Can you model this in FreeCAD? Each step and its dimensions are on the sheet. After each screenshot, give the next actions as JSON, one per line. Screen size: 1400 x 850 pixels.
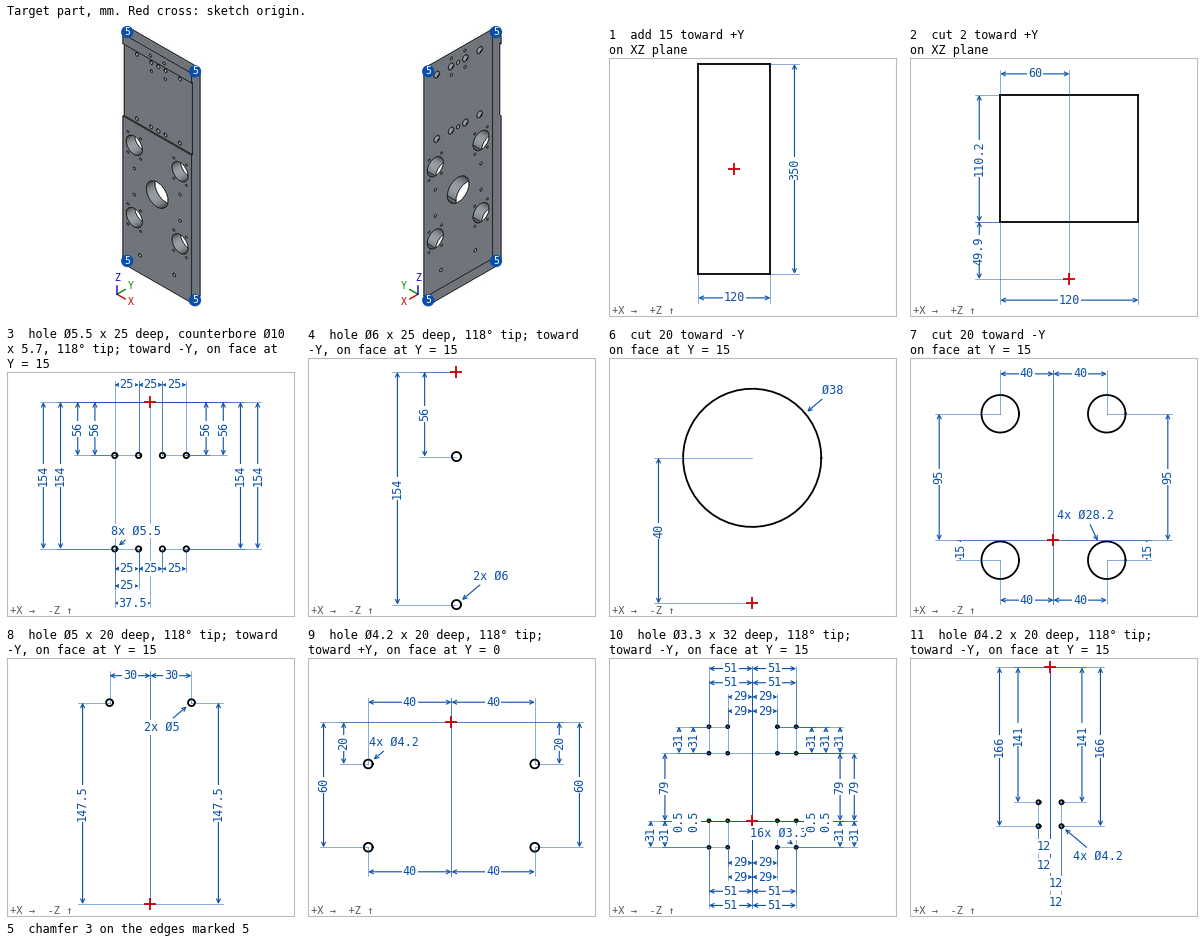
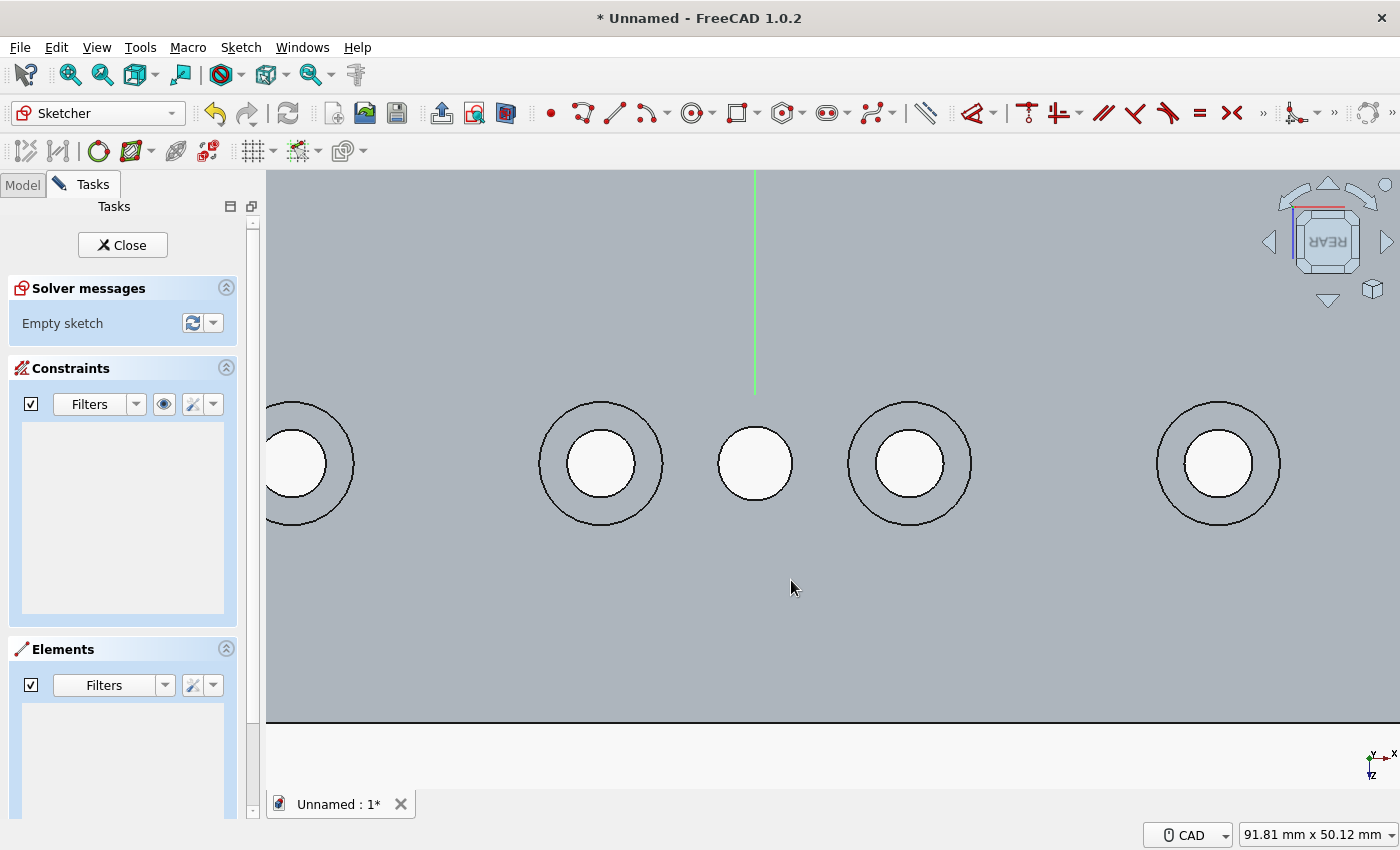
{"action": "left_click", "coordinate": [692, 114]}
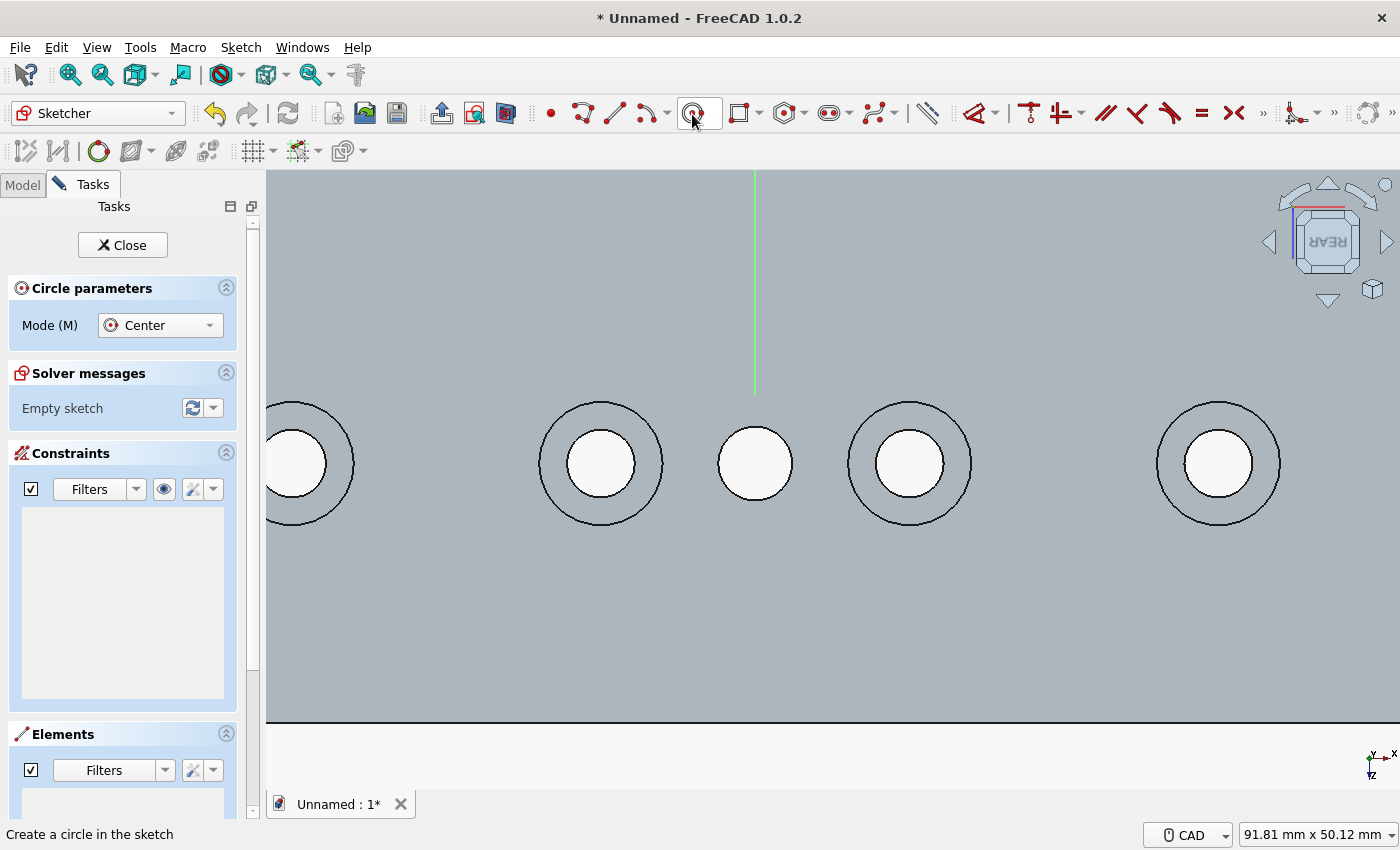
{"action": "left_click", "coordinate": [607, 303]}
{"action": "left_click", "coordinate": [625, 285]}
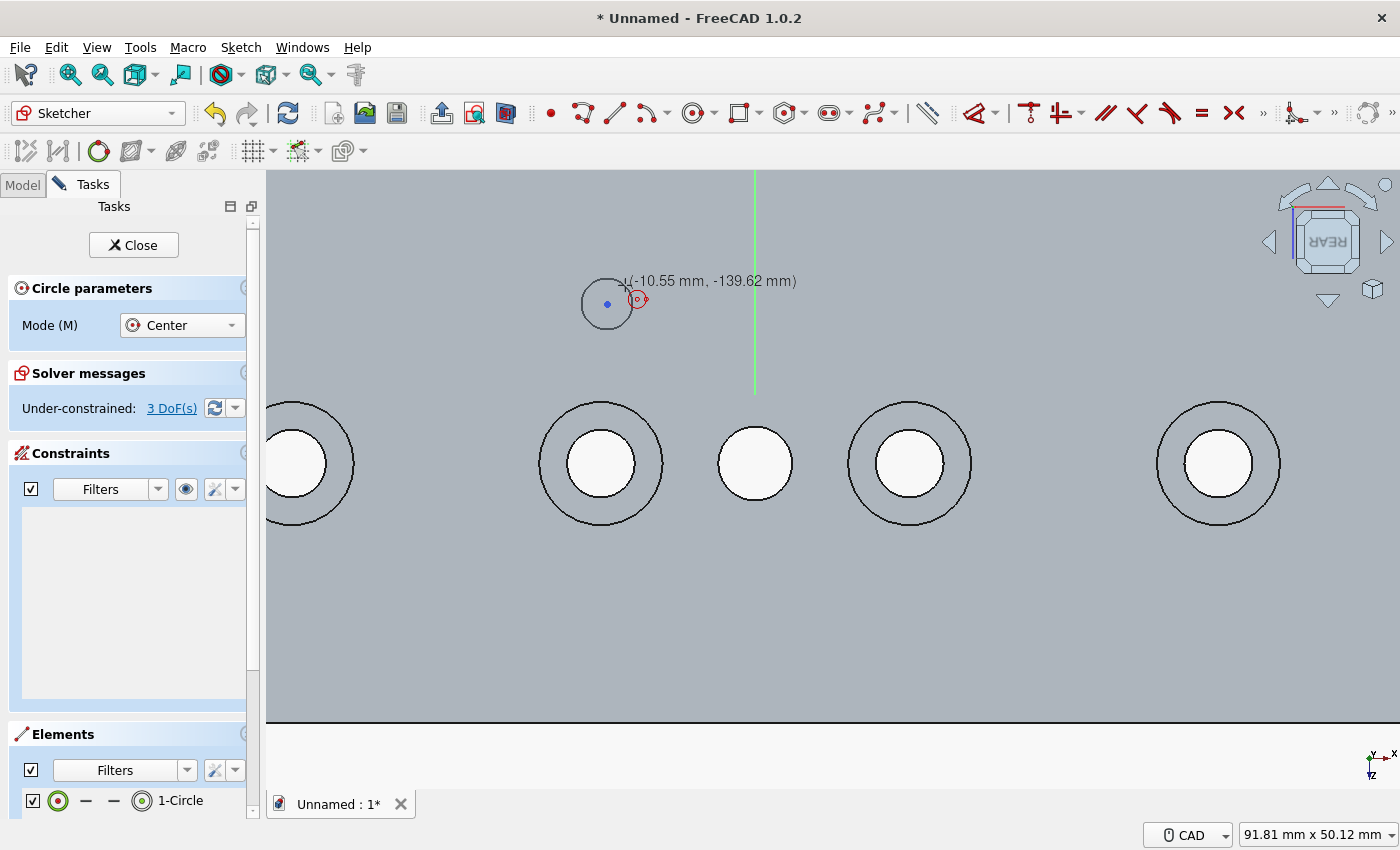
{"action": "left_click", "coordinate": [903, 303]}
{"action": "left_click", "coordinate": [922, 285]}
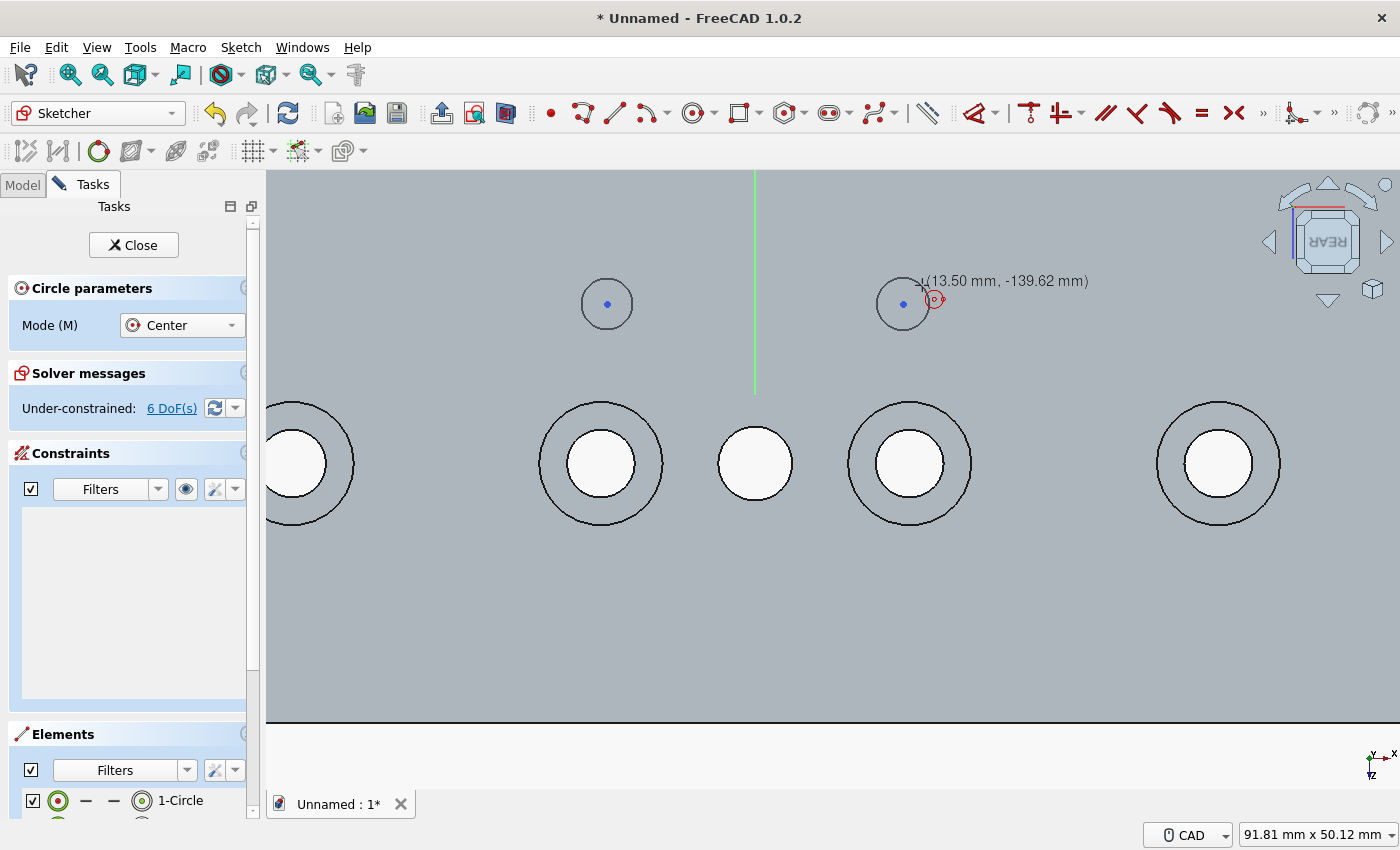
{"action": "left_click", "coordinate": [607, 612]}
{"action": "left_click", "coordinate": [625, 593]}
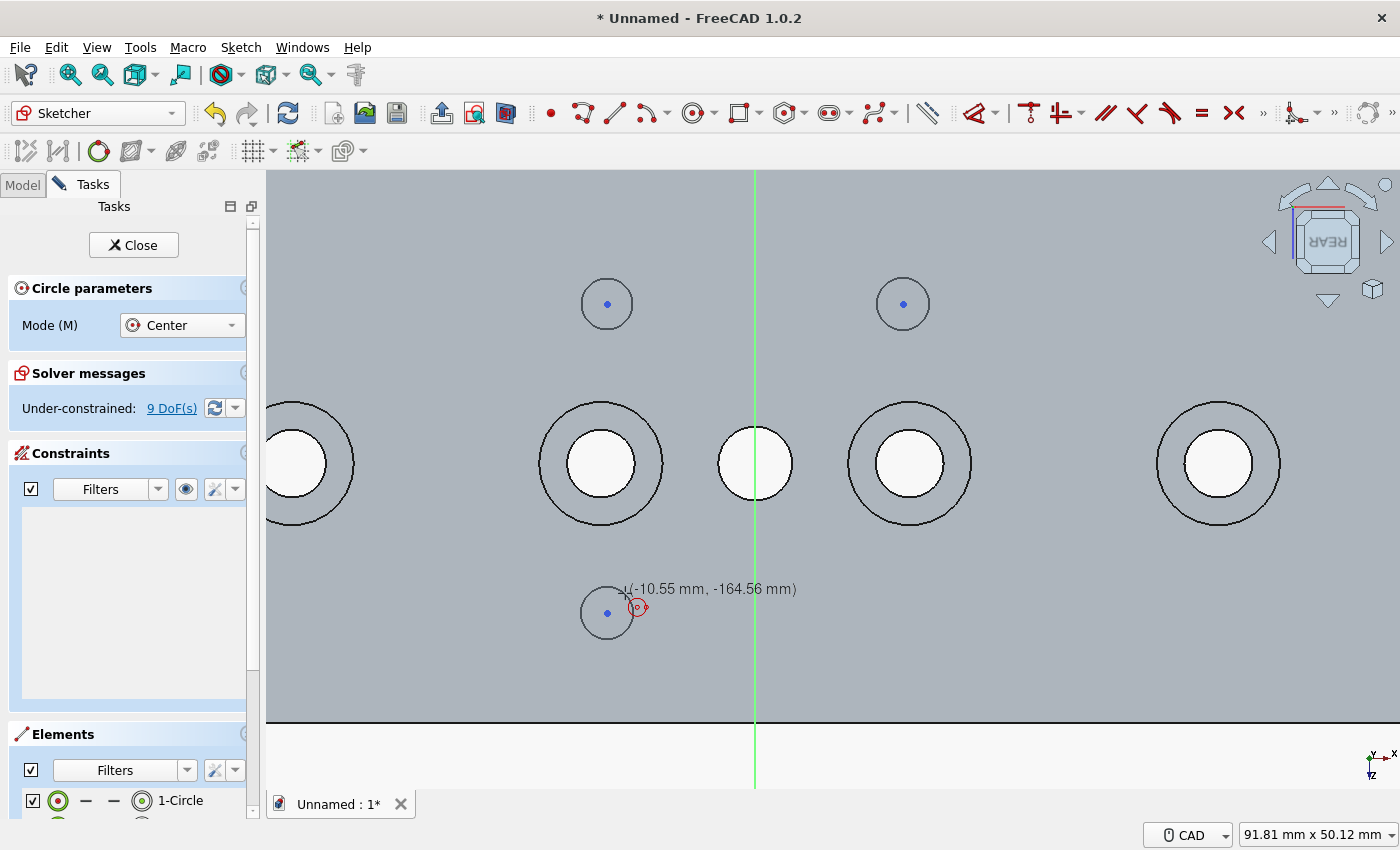
{"action": "left_click", "coordinate": [903, 612]}
{"action": "left_click", "coordinate": [922, 593]}
{"action": "key", "text": "Escape"}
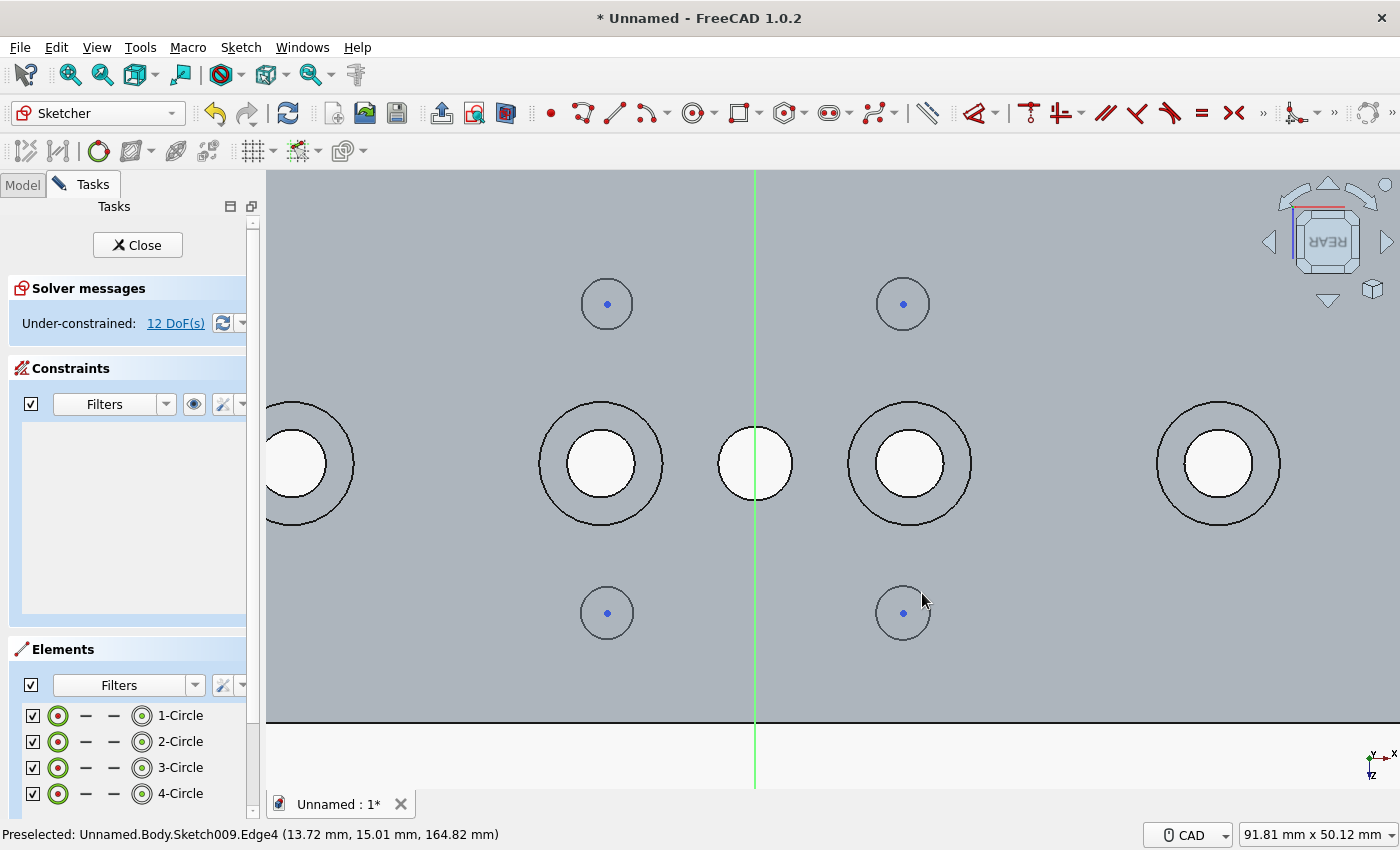
{"action": "left_click", "coordinate": [625, 286]}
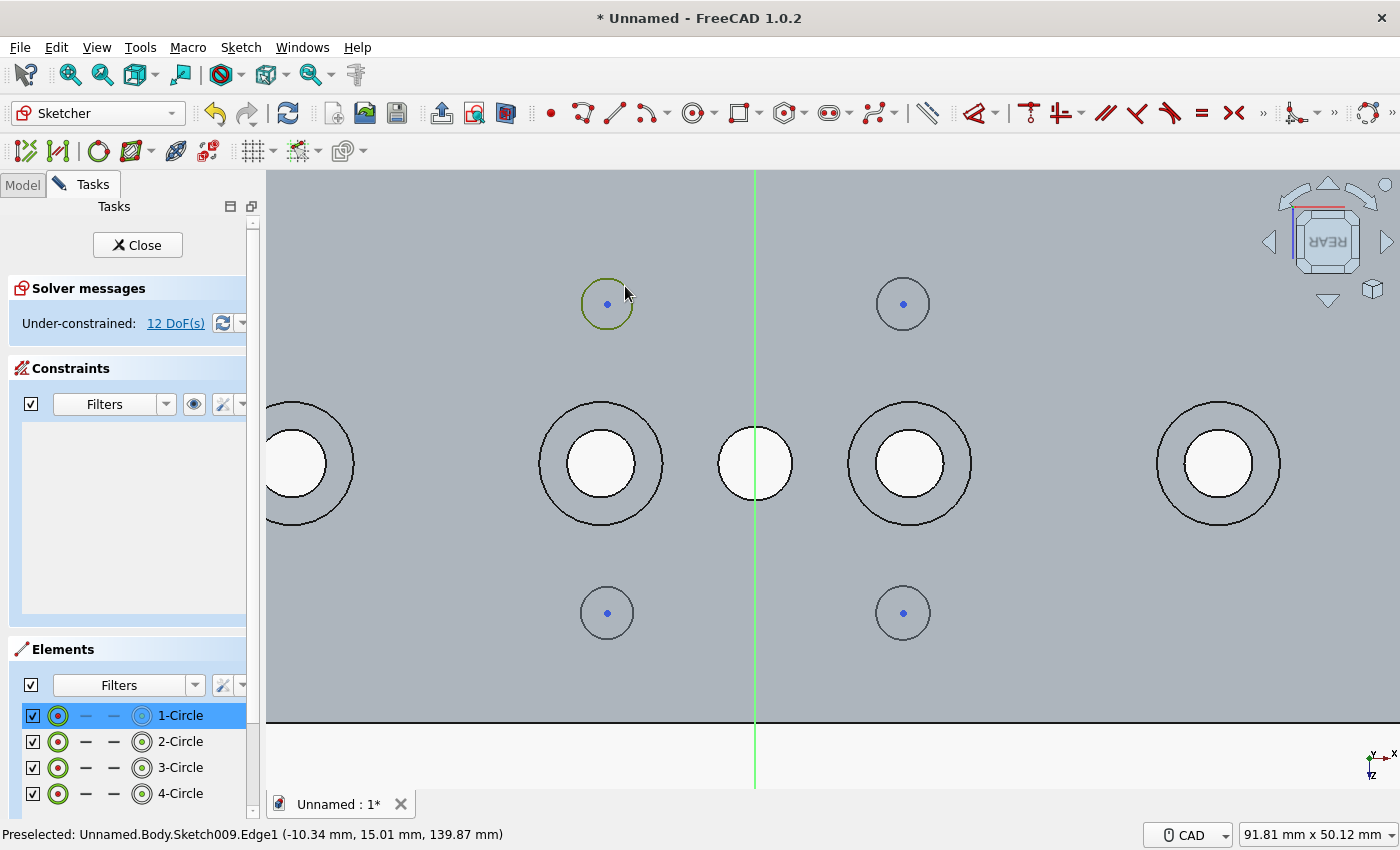
{"action": "left_click", "coordinate": [921, 285]}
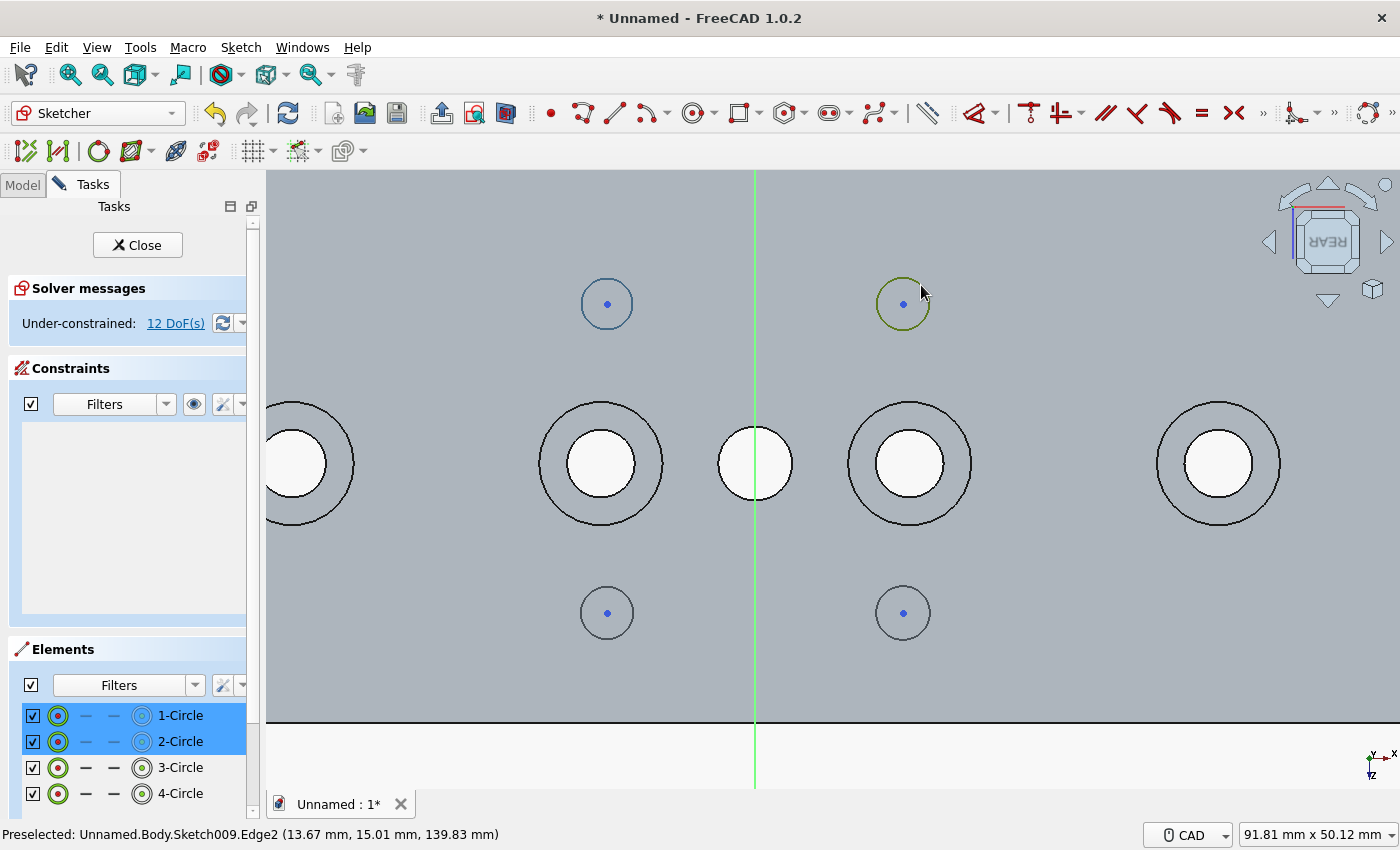
{"action": "left_click", "coordinate": [625, 594]}